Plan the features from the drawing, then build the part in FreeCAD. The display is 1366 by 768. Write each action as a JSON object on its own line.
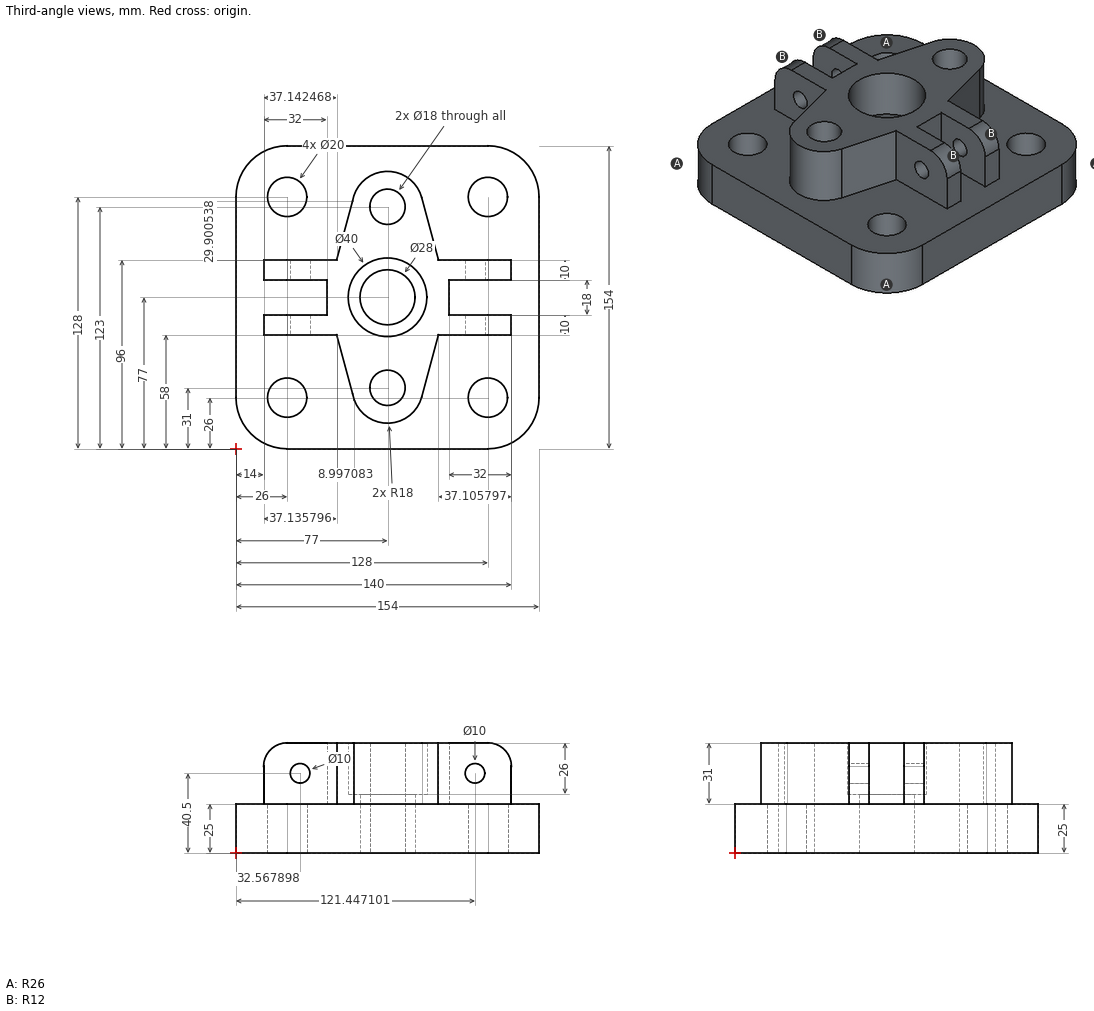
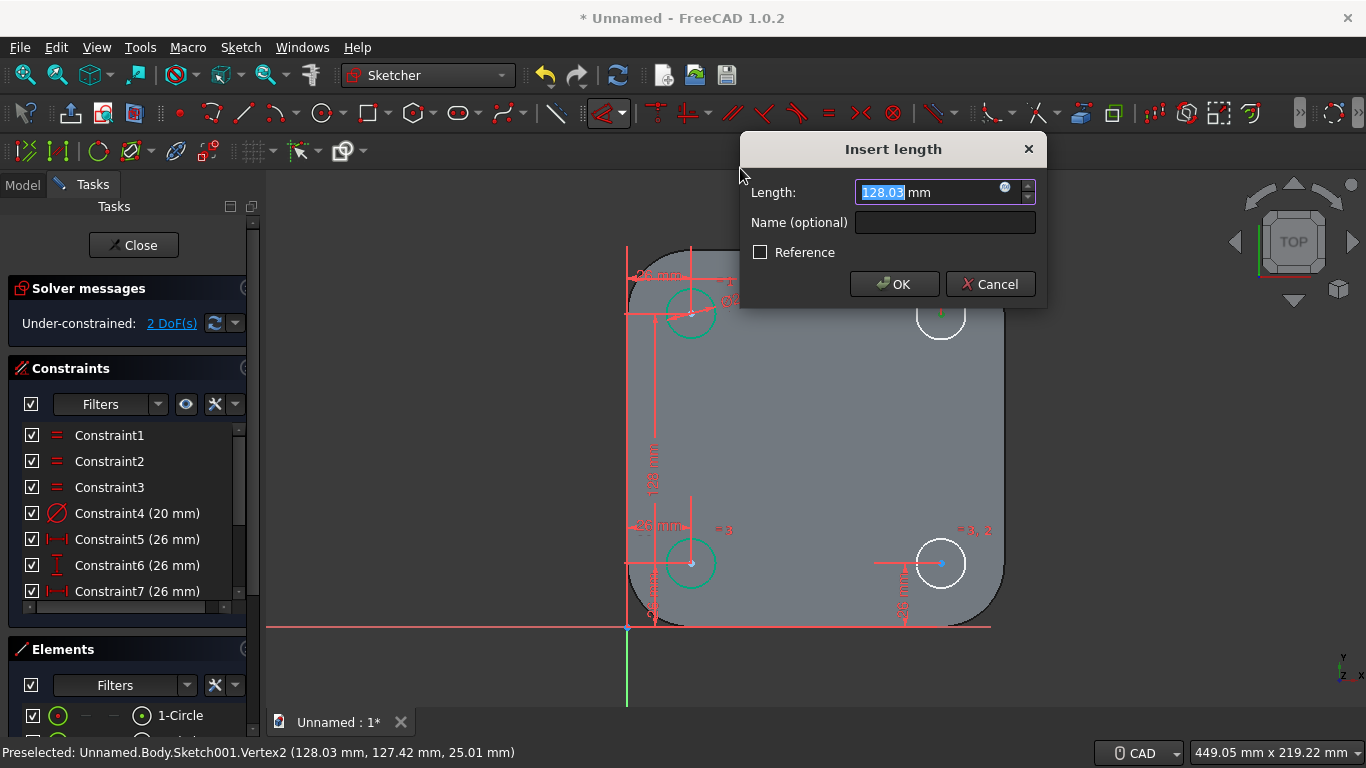
{"action": "type", "text": "128"}
{"action": "key", "text": "Return"}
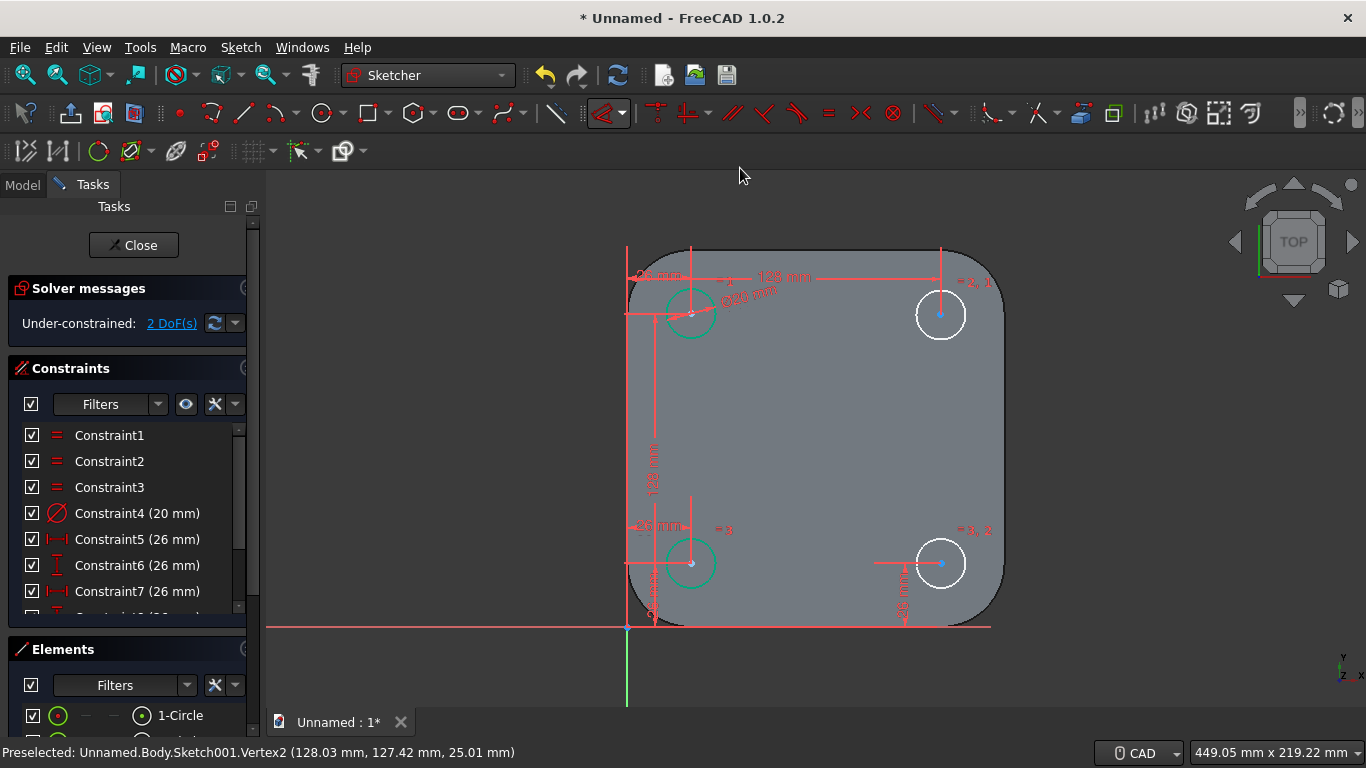
{"action": "left_click", "coordinate": [941, 315]}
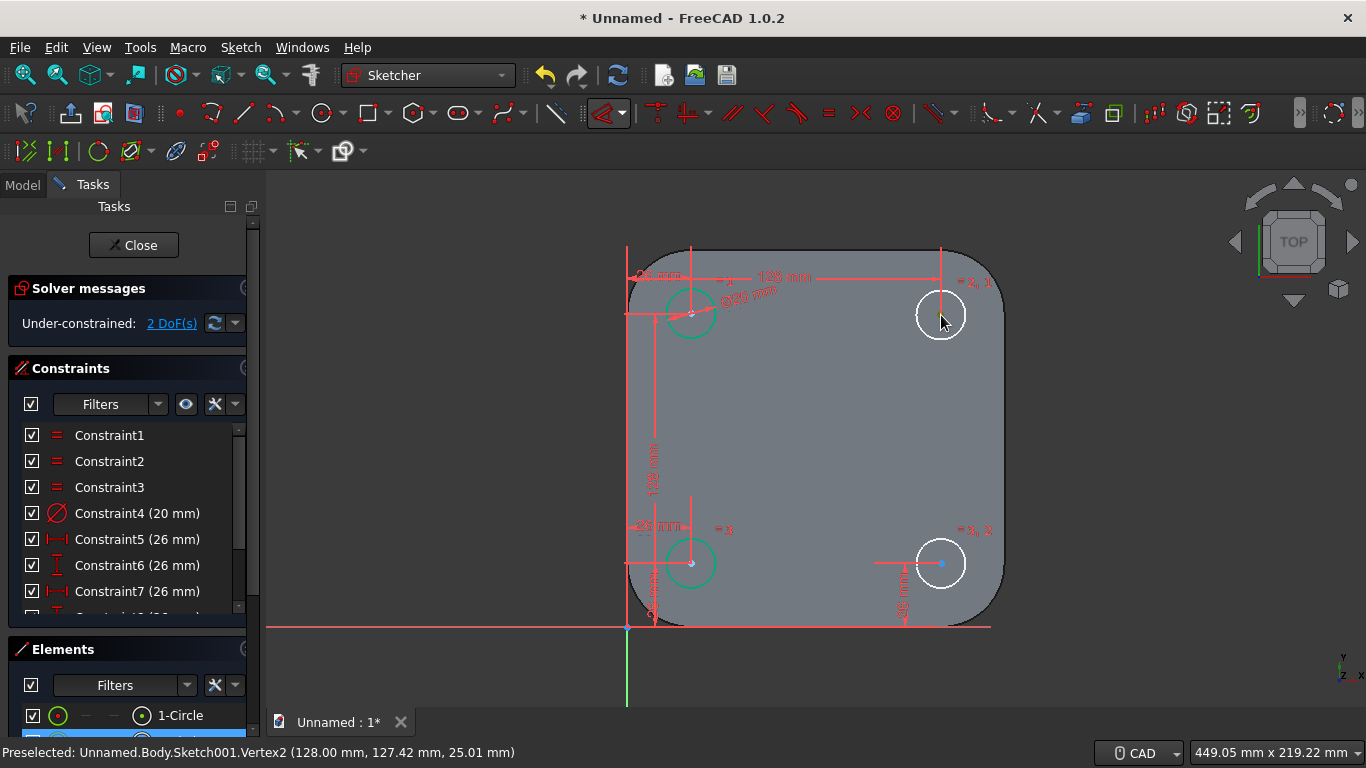
{"action": "left_click", "coordinate": [624, 114]}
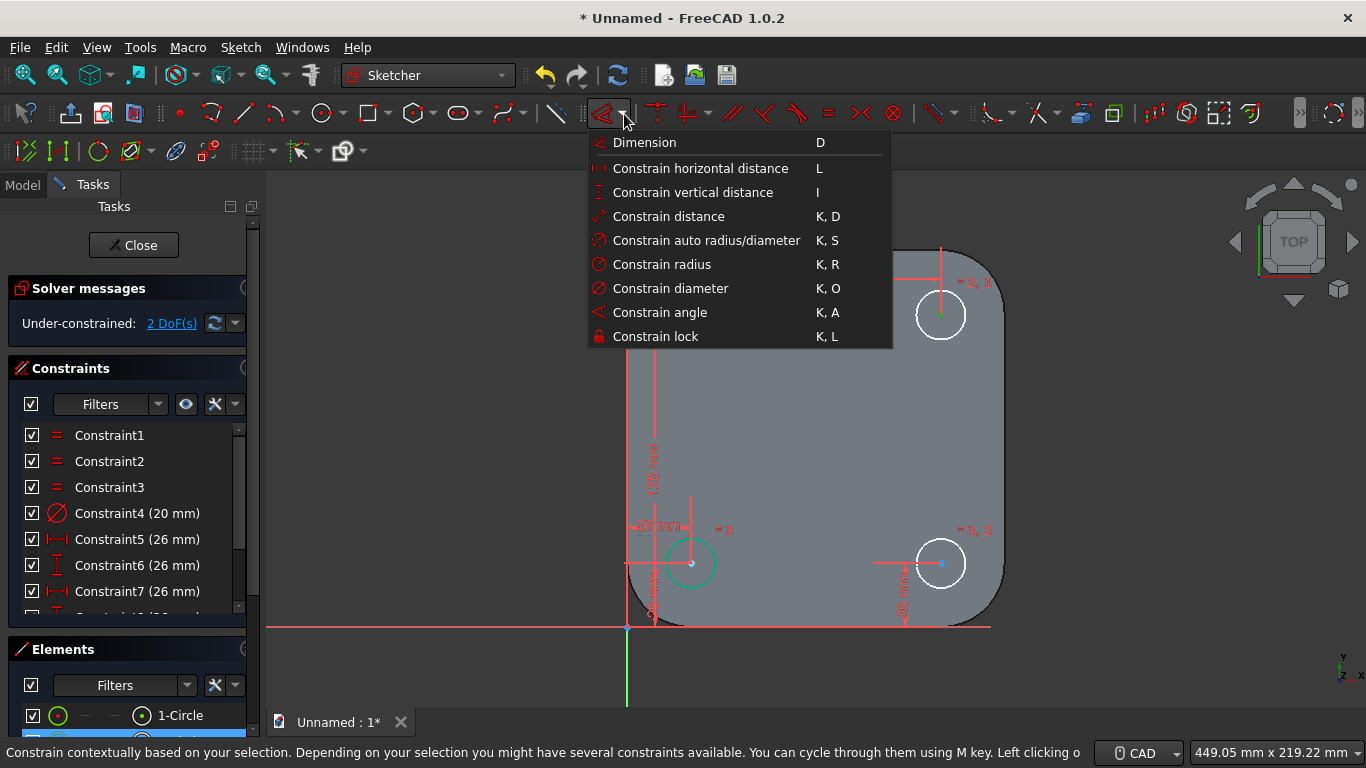
{"action": "left_click", "coordinate": [740, 192]}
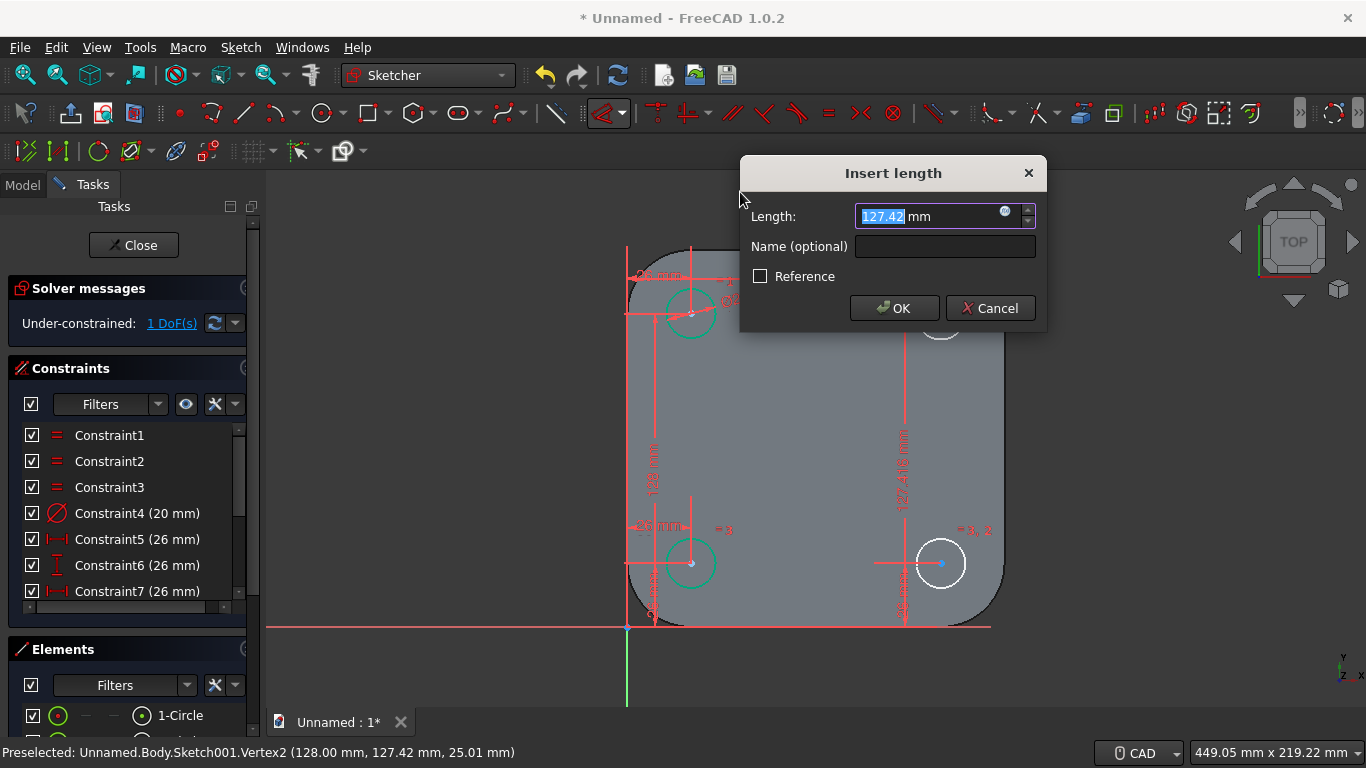
{"action": "type", "text": "128"}
{"action": "key", "text": "Return"}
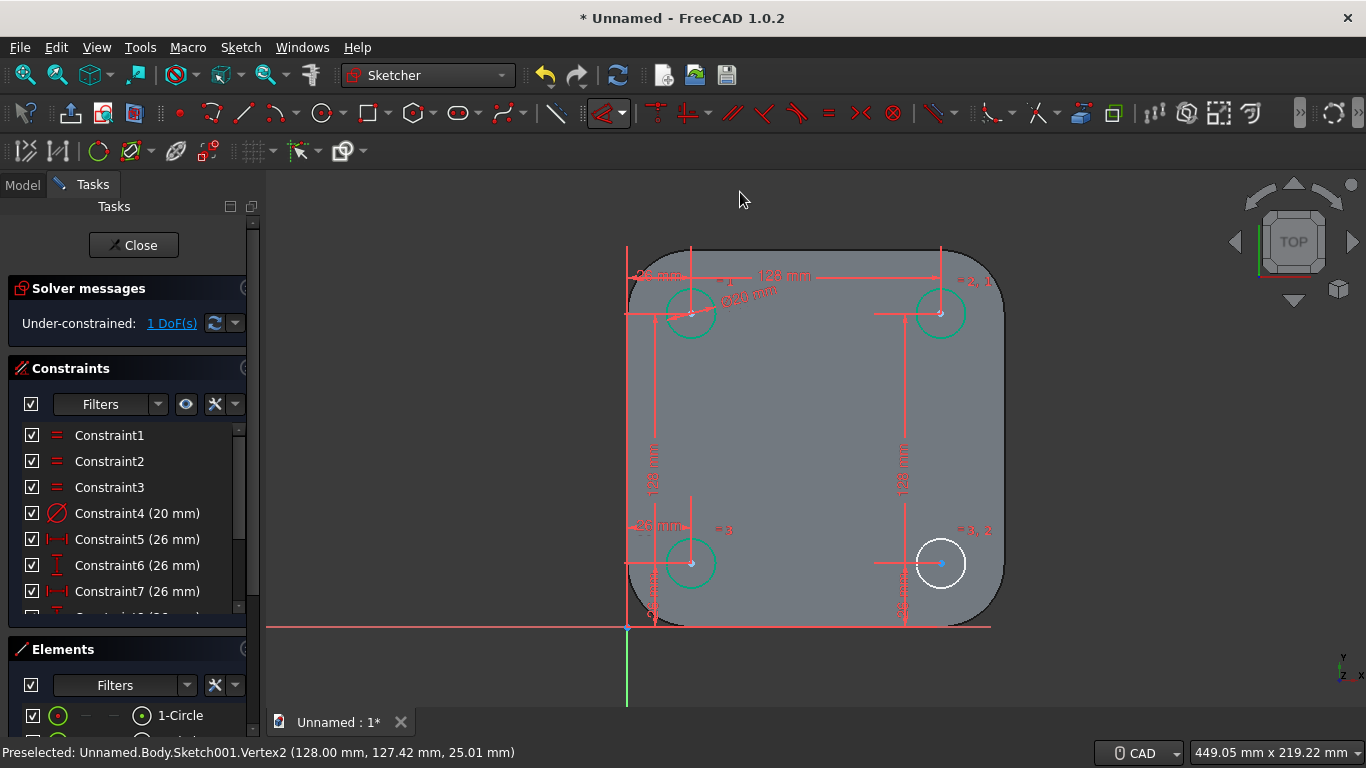
{"action": "left_click", "coordinate": [941, 563]}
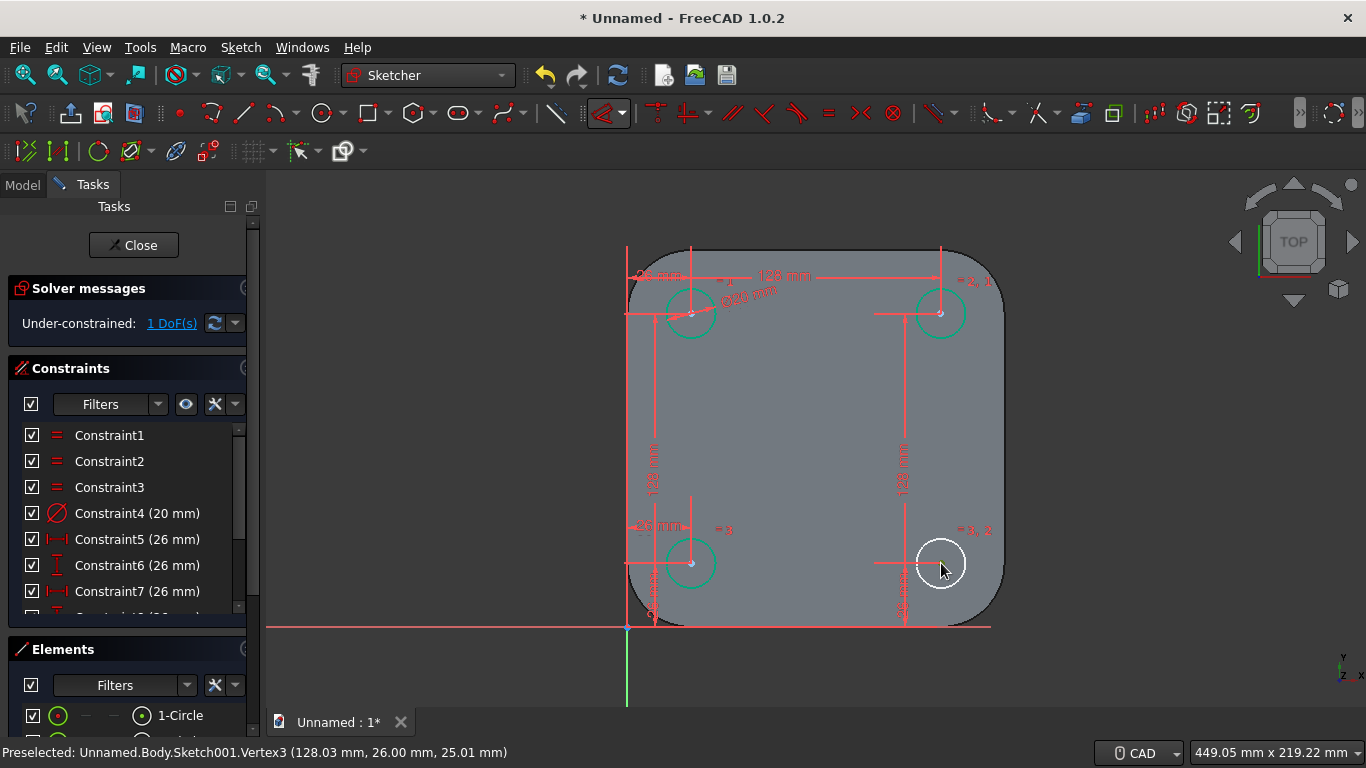
{"action": "left_click", "coordinate": [624, 114]}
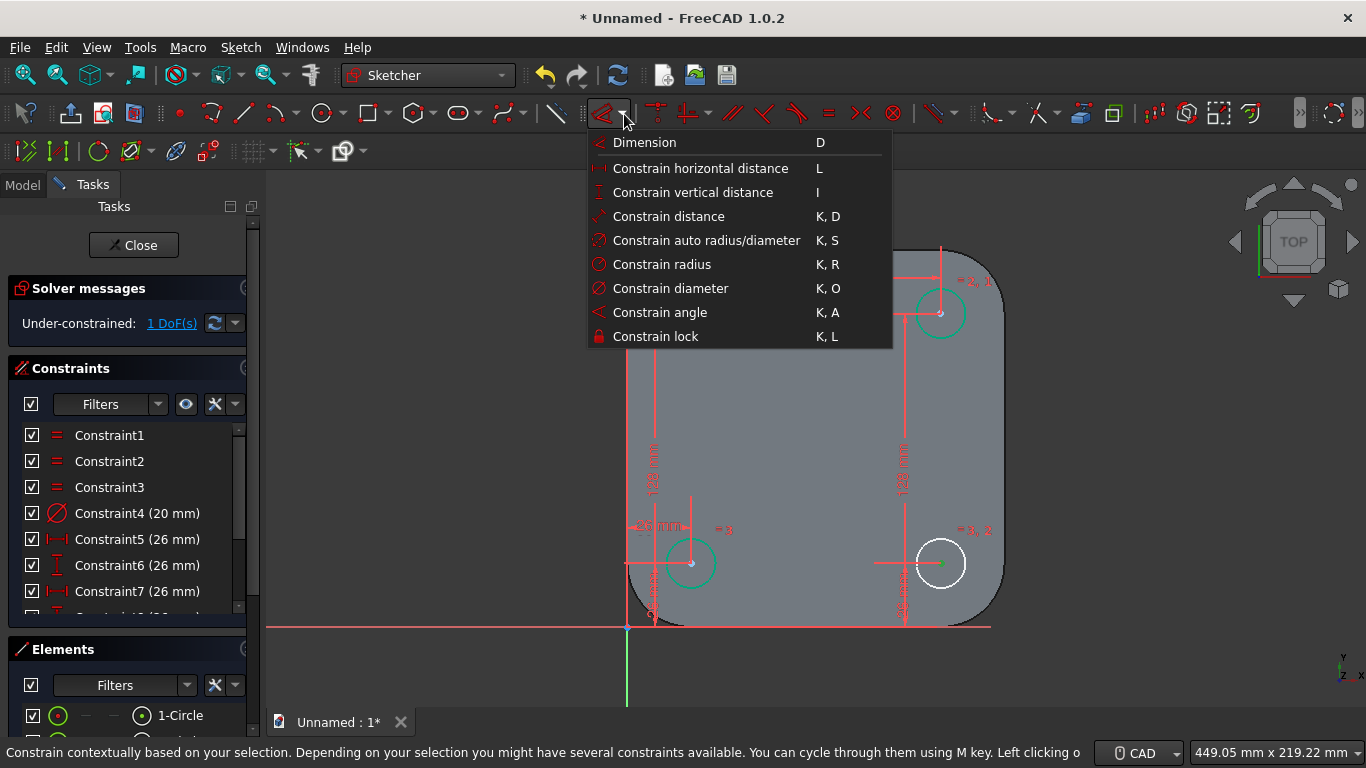
{"action": "left_click", "coordinate": [740, 168]}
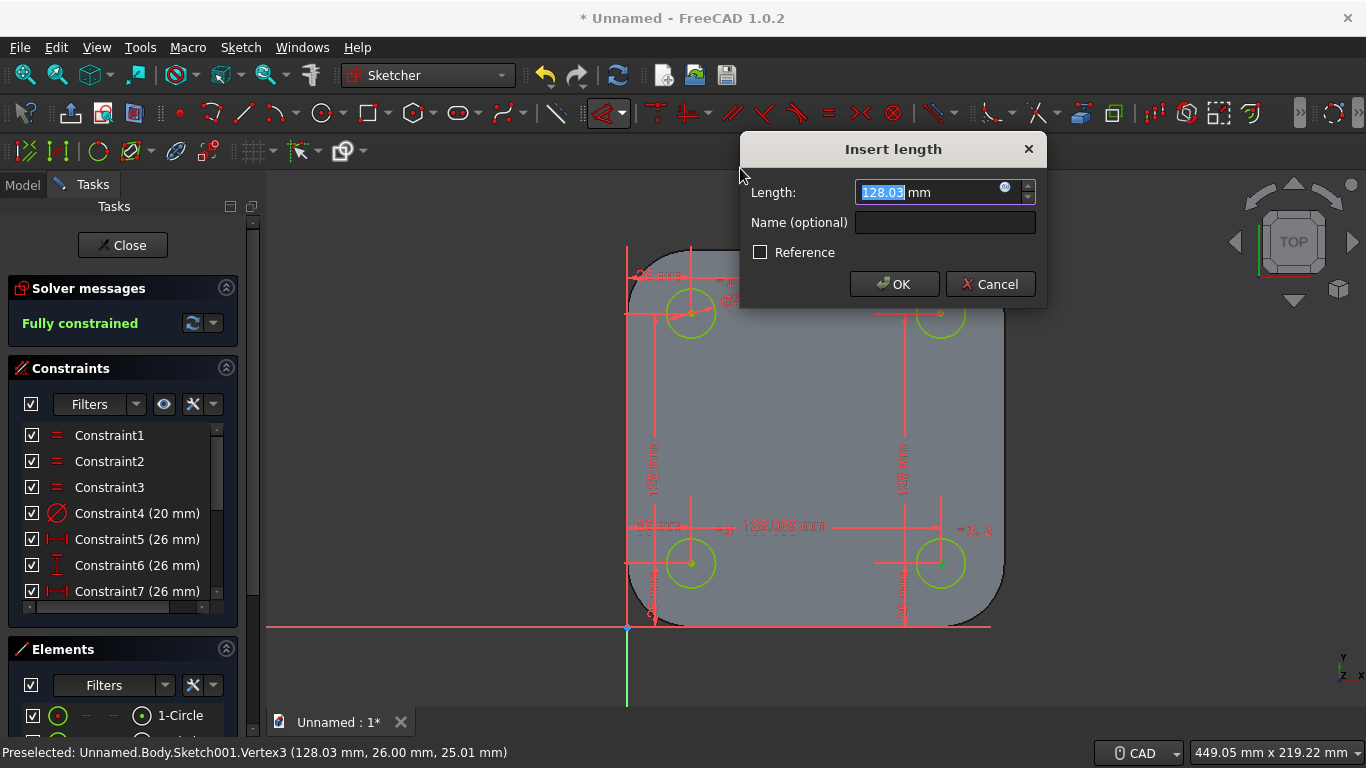
{"action": "type", "text": "128"}
{"action": "key", "text": "Return"}